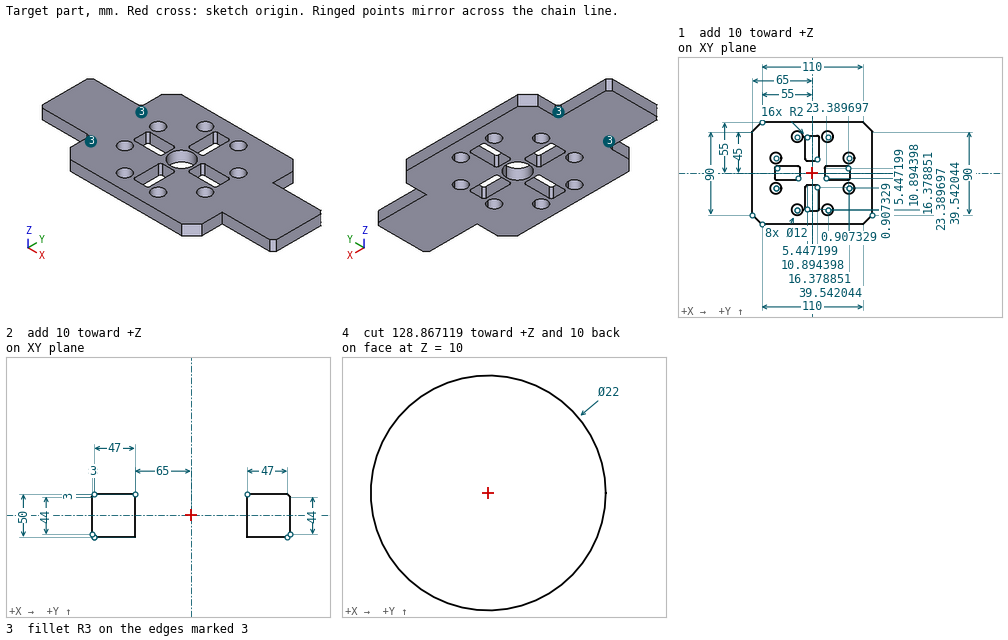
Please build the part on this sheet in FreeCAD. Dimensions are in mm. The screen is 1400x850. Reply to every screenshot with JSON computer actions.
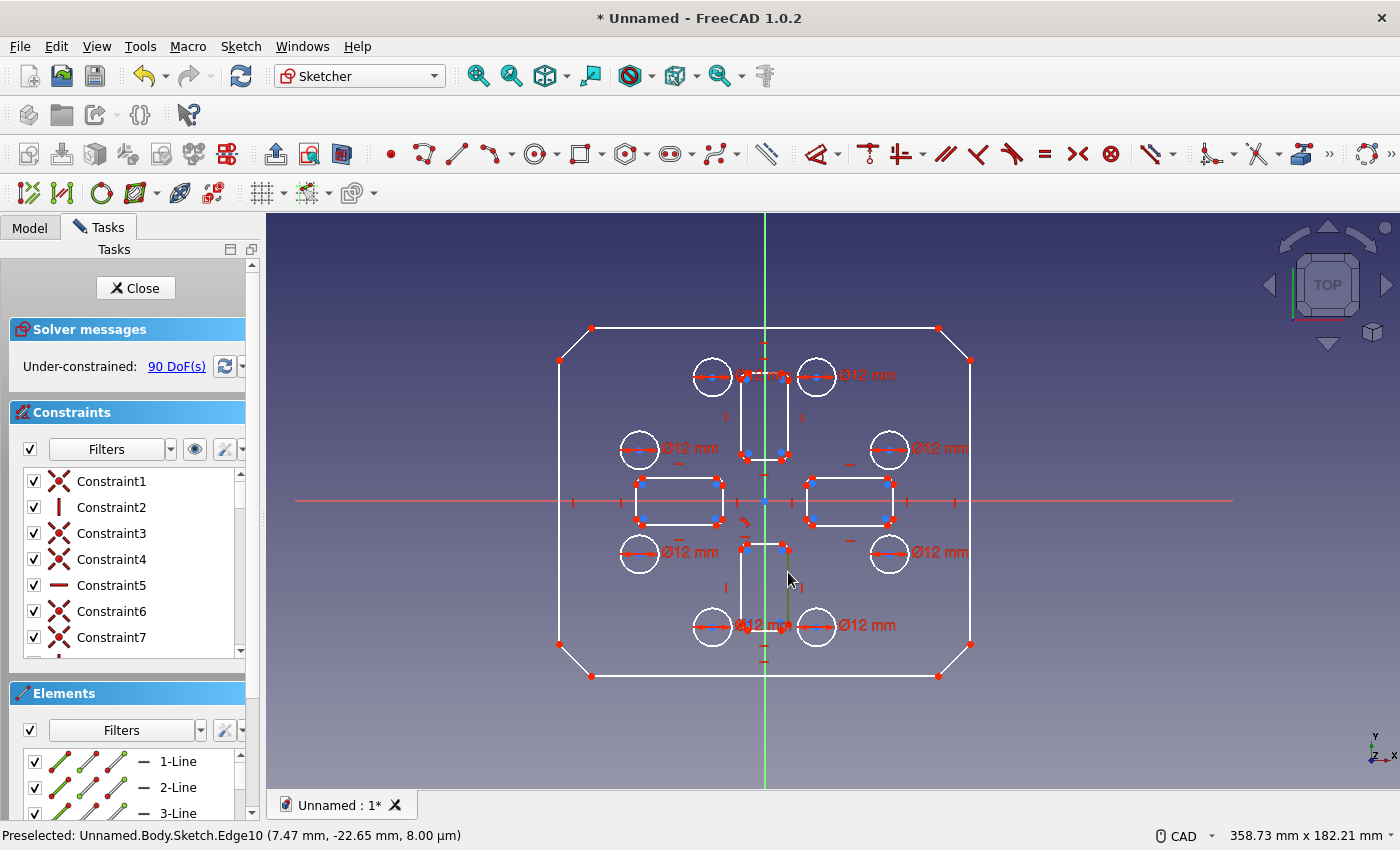
{"action": "scroll", "coordinate": [786, 546], "scroll_direction": "up", "scroll_amount": 6}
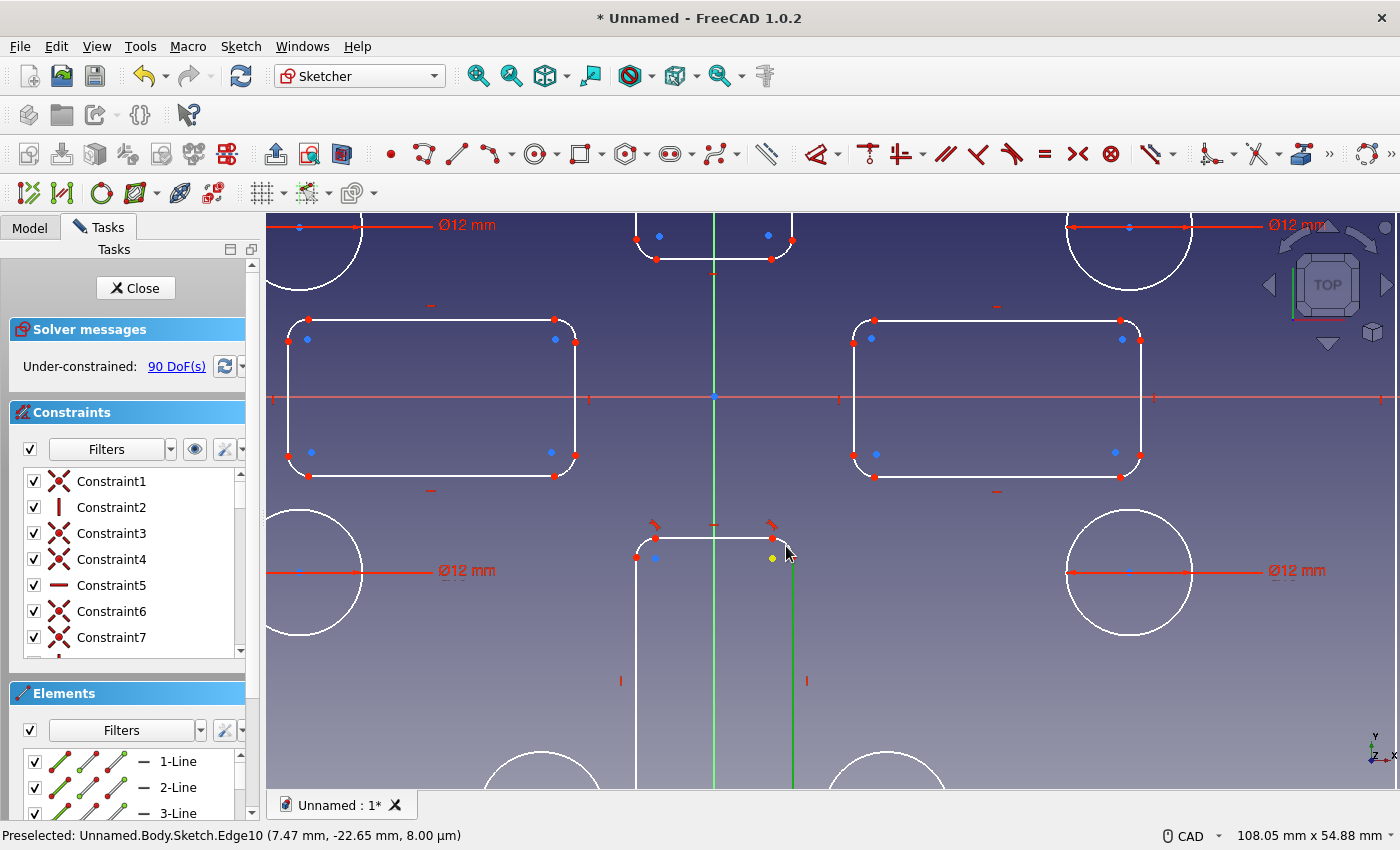
{"action": "left_click", "coordinate": [787, 544]}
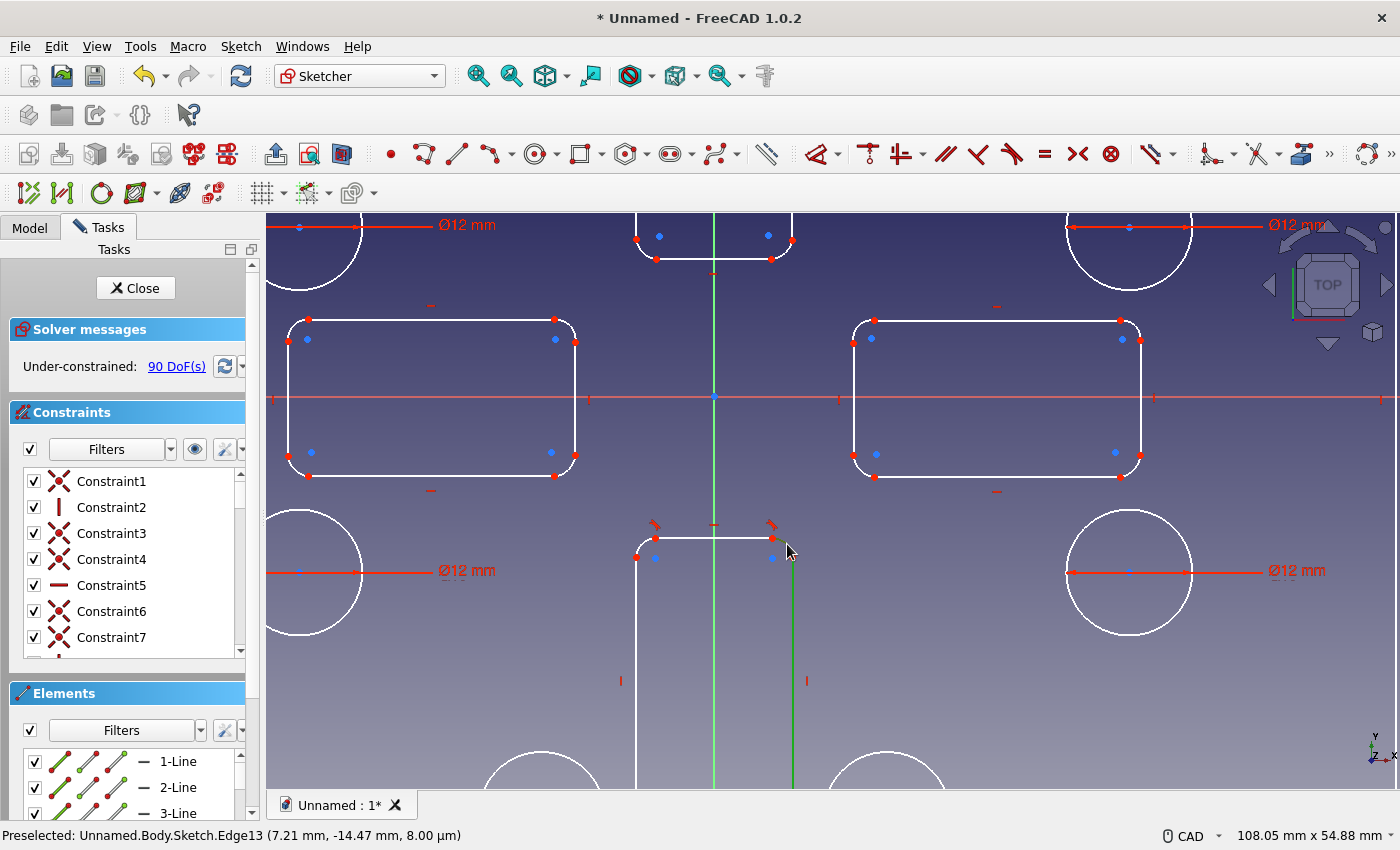
{"action": "left_click", "coordinate": [1012, 154]}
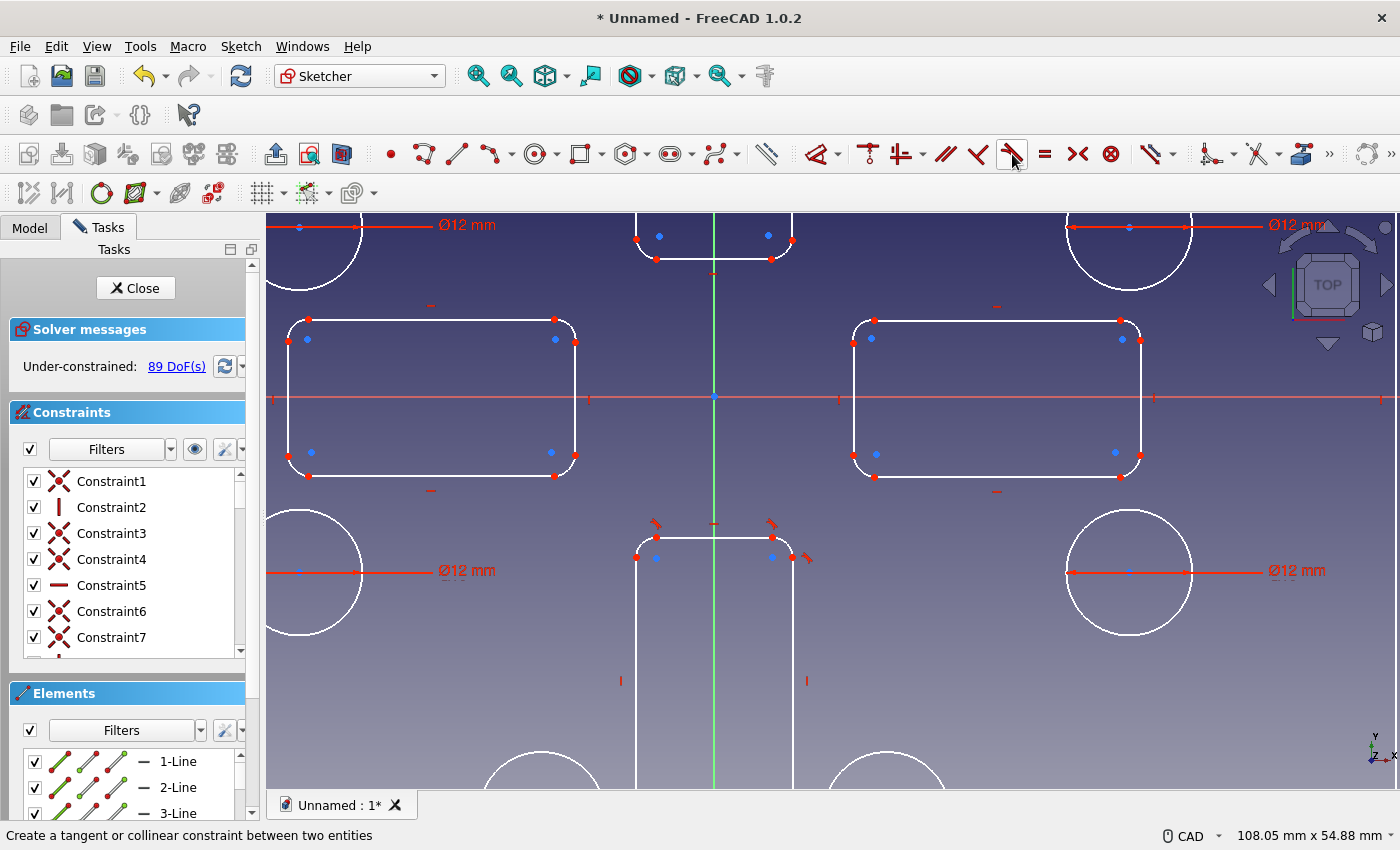
{"action": "left_click", "coordinate": [793, 632]}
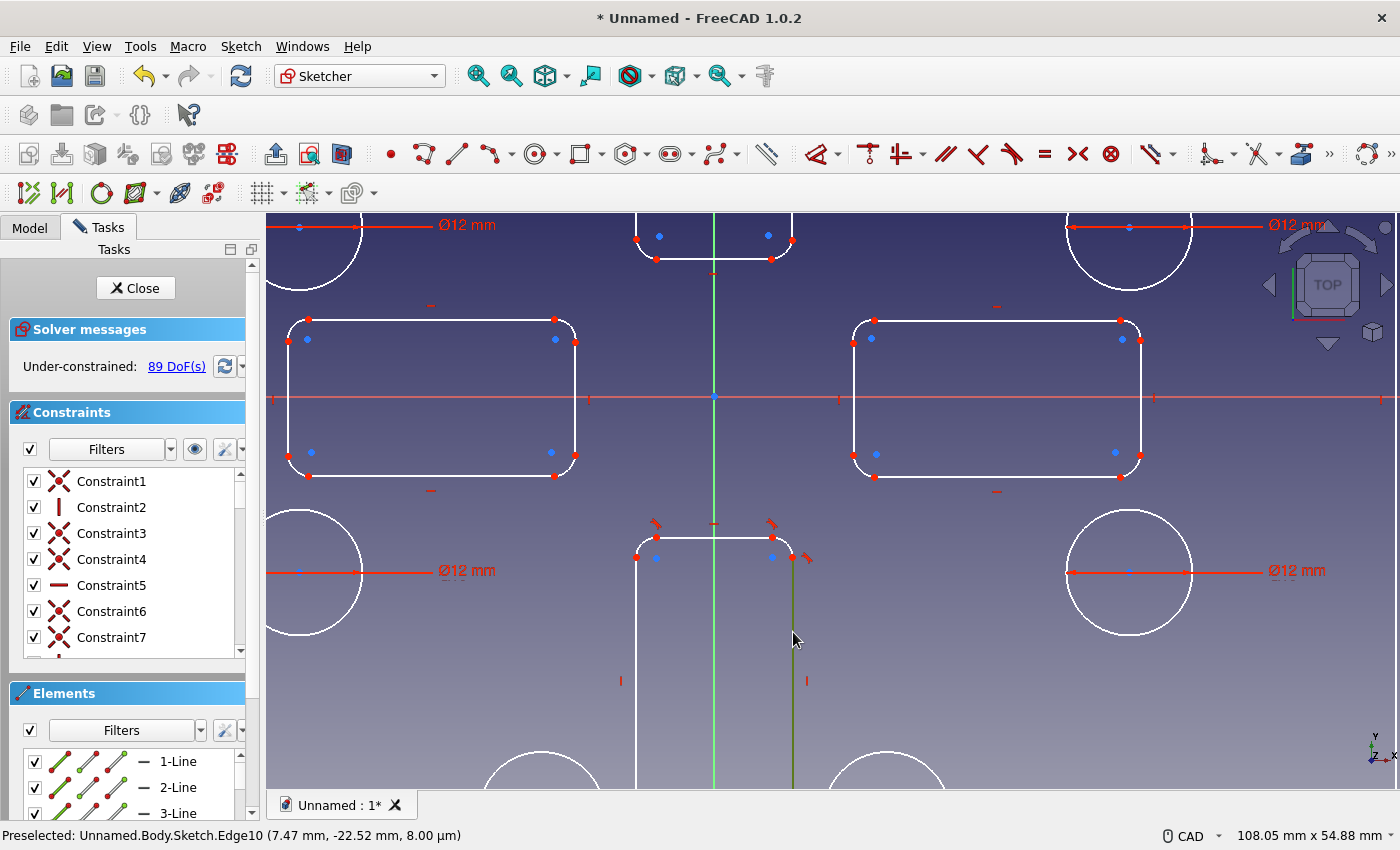
{"action": "scroll", "coordinate": [786, 546], "scroll_direction": "down", "scroll_amount": 6}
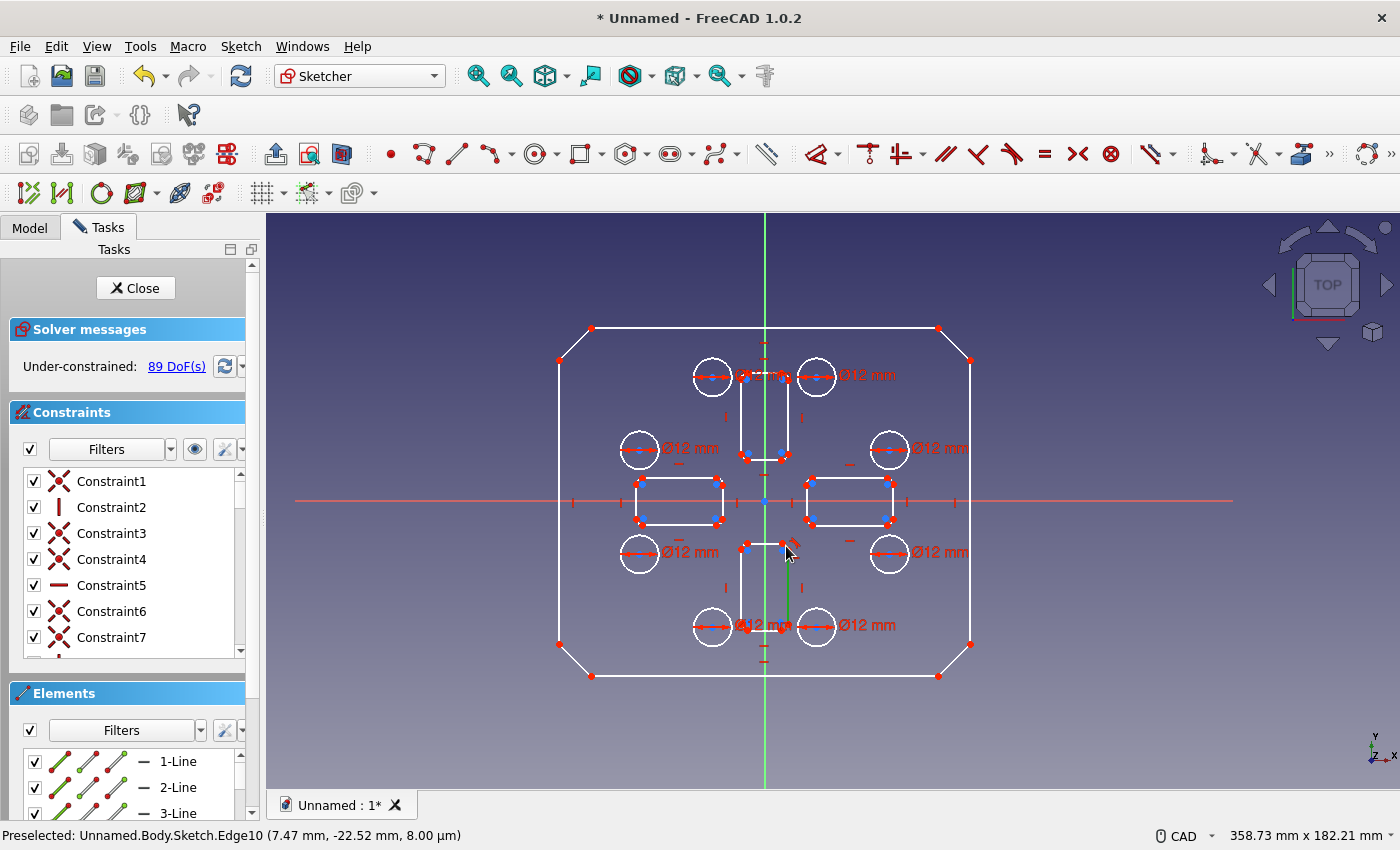
{"action": "scroll", "coordinate": [785, 630], "scroll_direction": "up", "scroll_amount": 8}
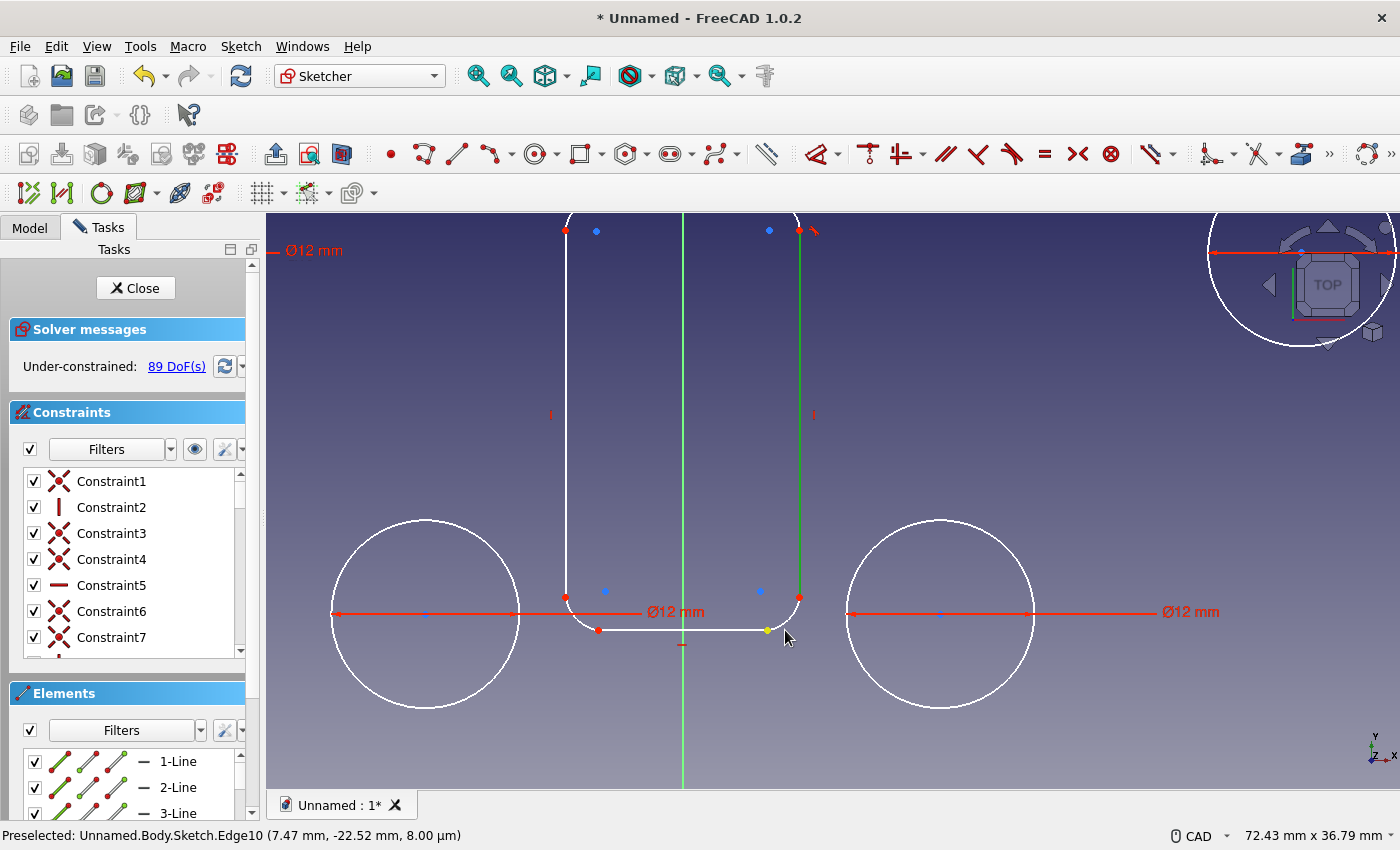
{"action": "left_click", "coordinate": [781, 625]}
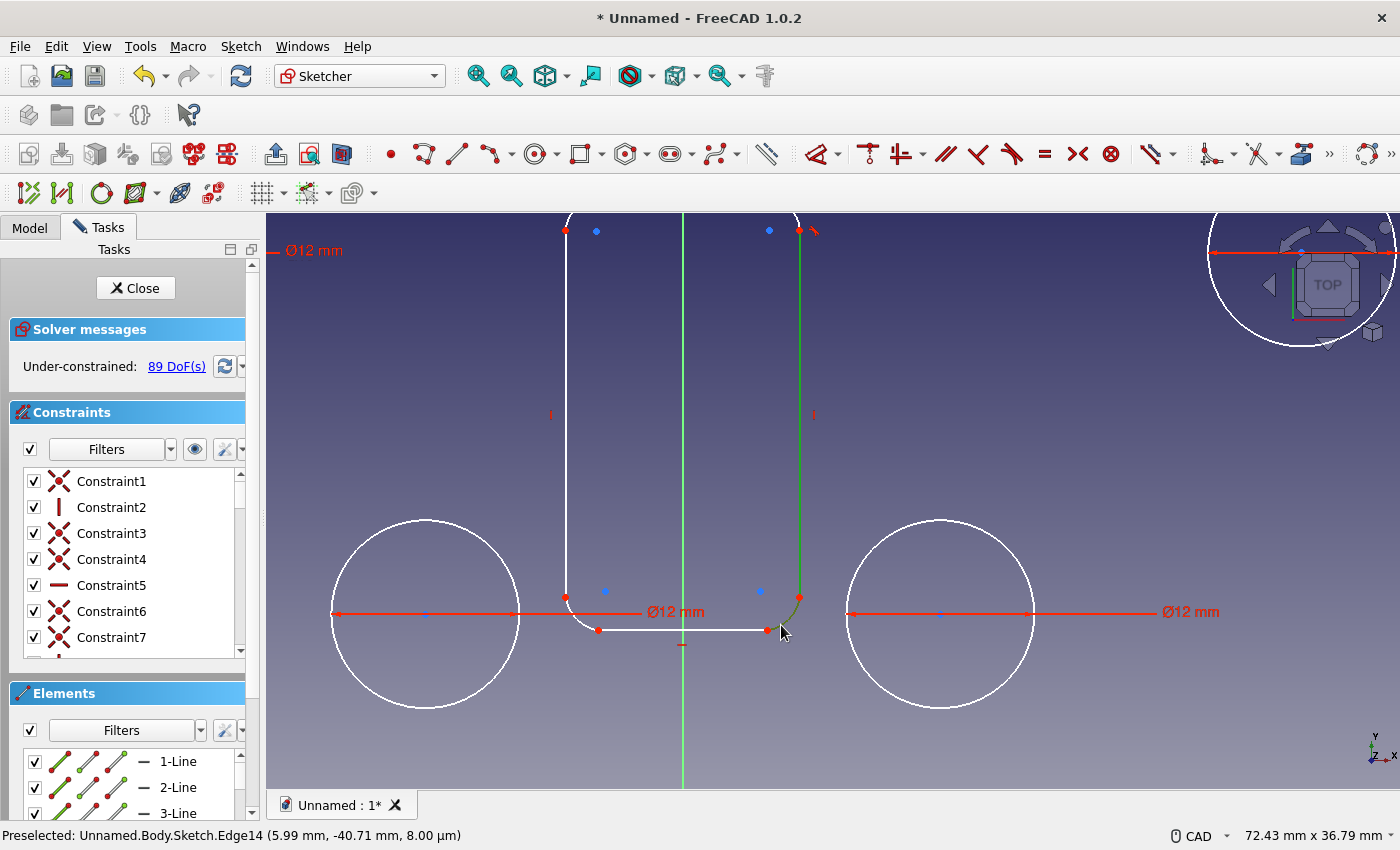
{"action": "left_click", "coordinate": [1012, 154]}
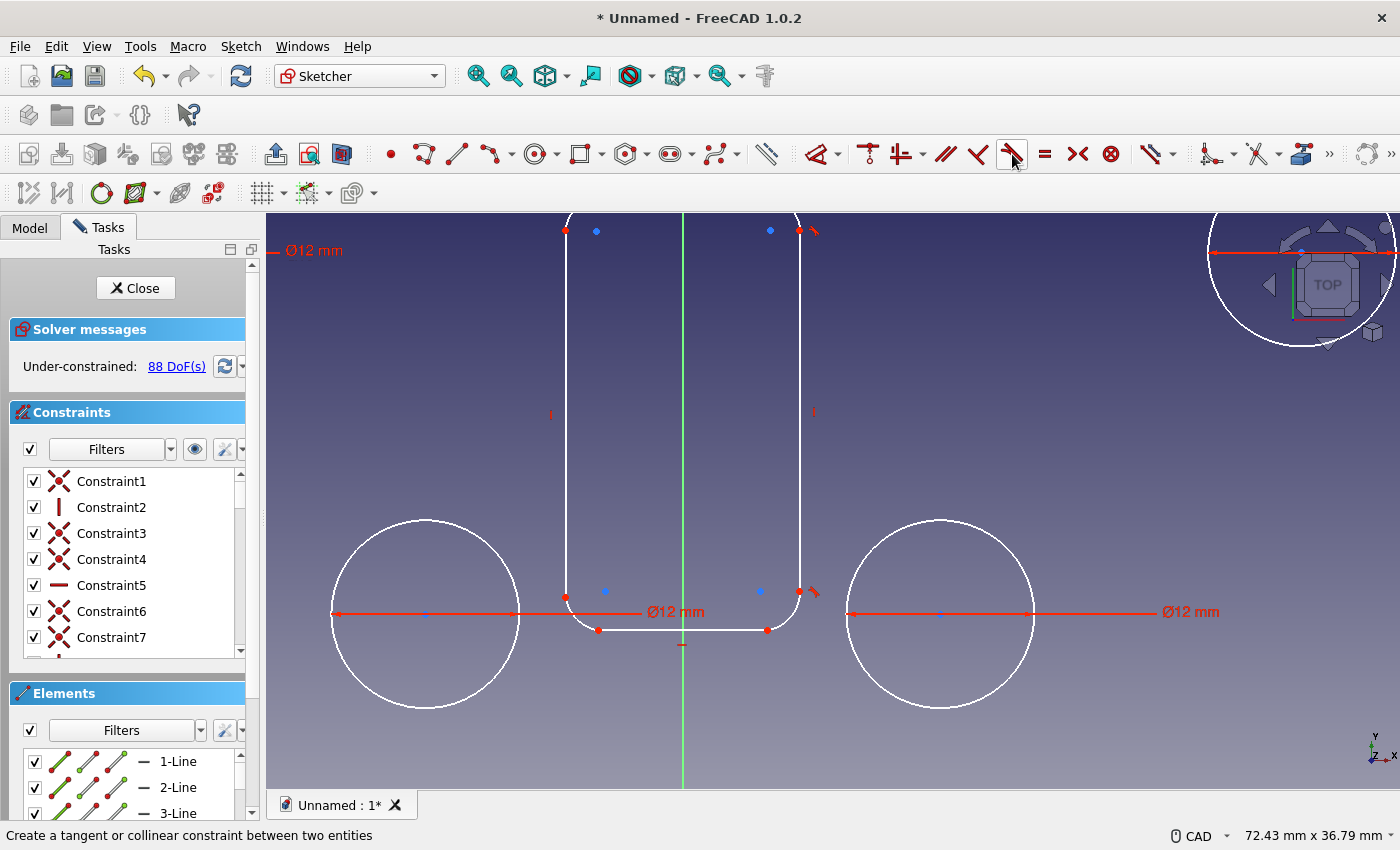
{"action": "left_click", "coordinate": [717, 630]}